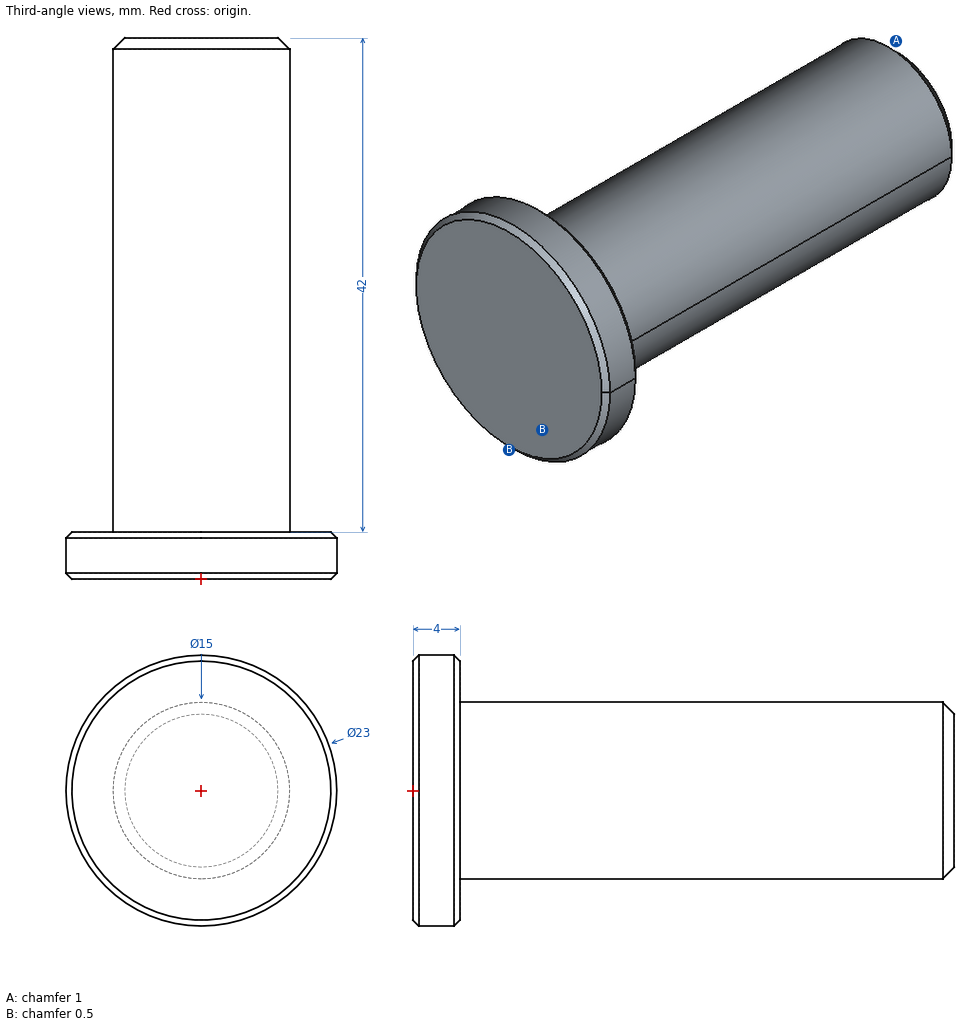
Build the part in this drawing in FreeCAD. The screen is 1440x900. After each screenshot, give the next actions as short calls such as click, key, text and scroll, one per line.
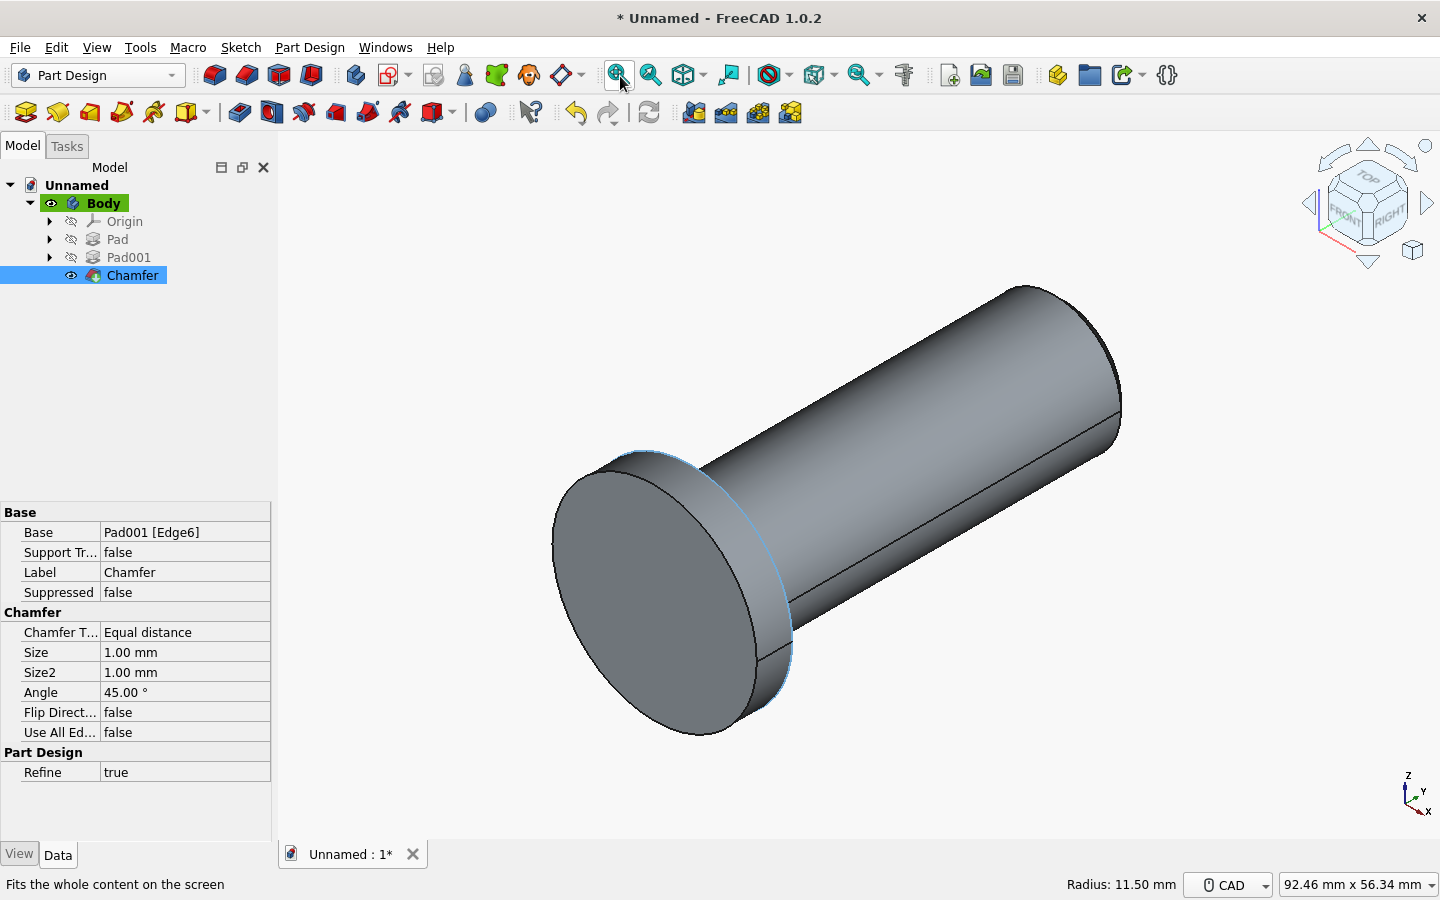
click(623, 472, ctrl)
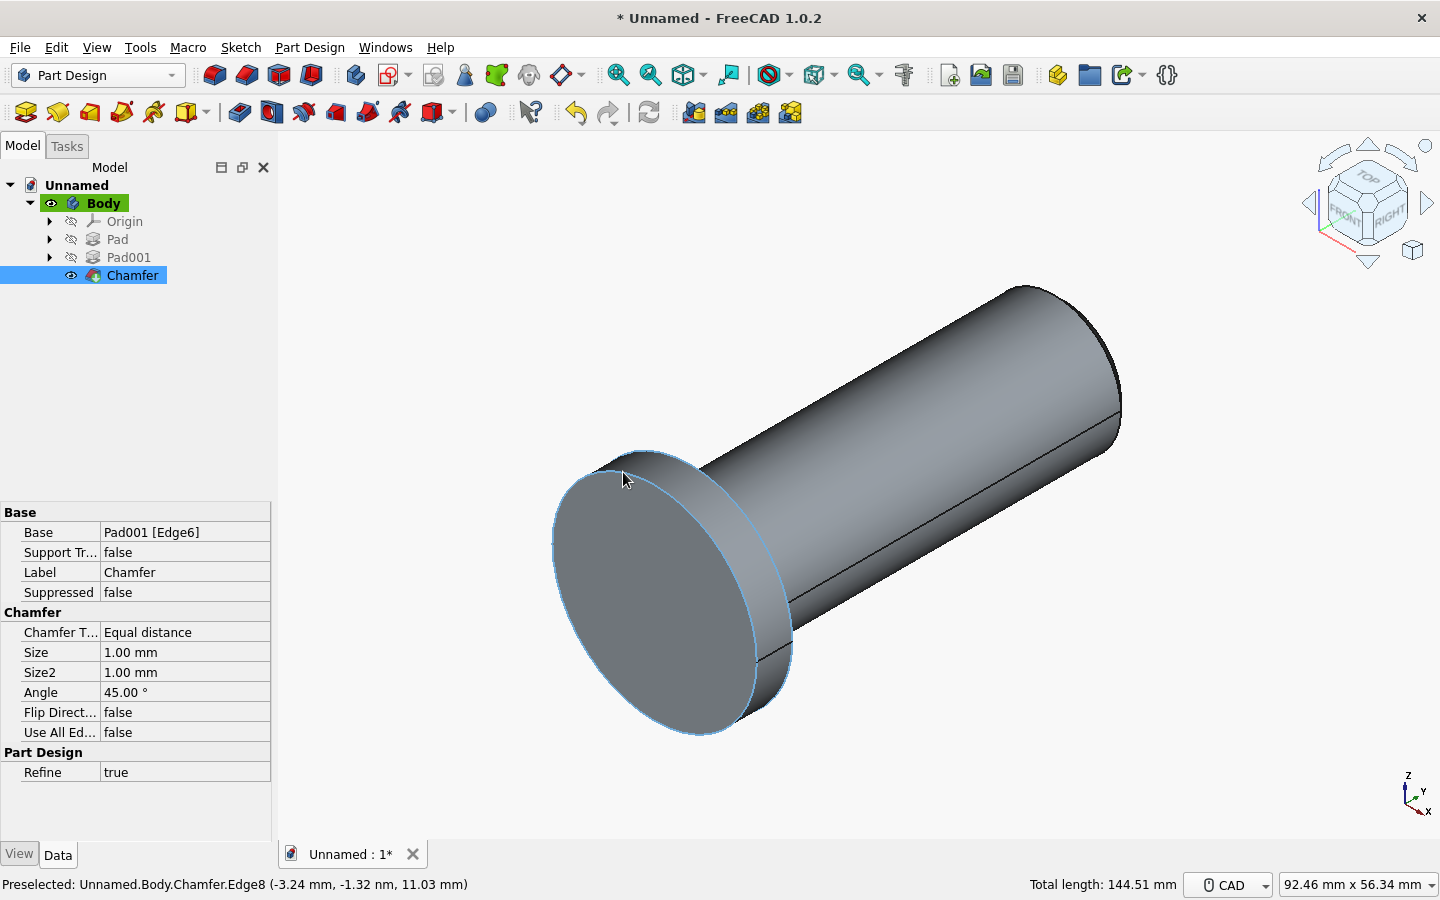
click(248, 76)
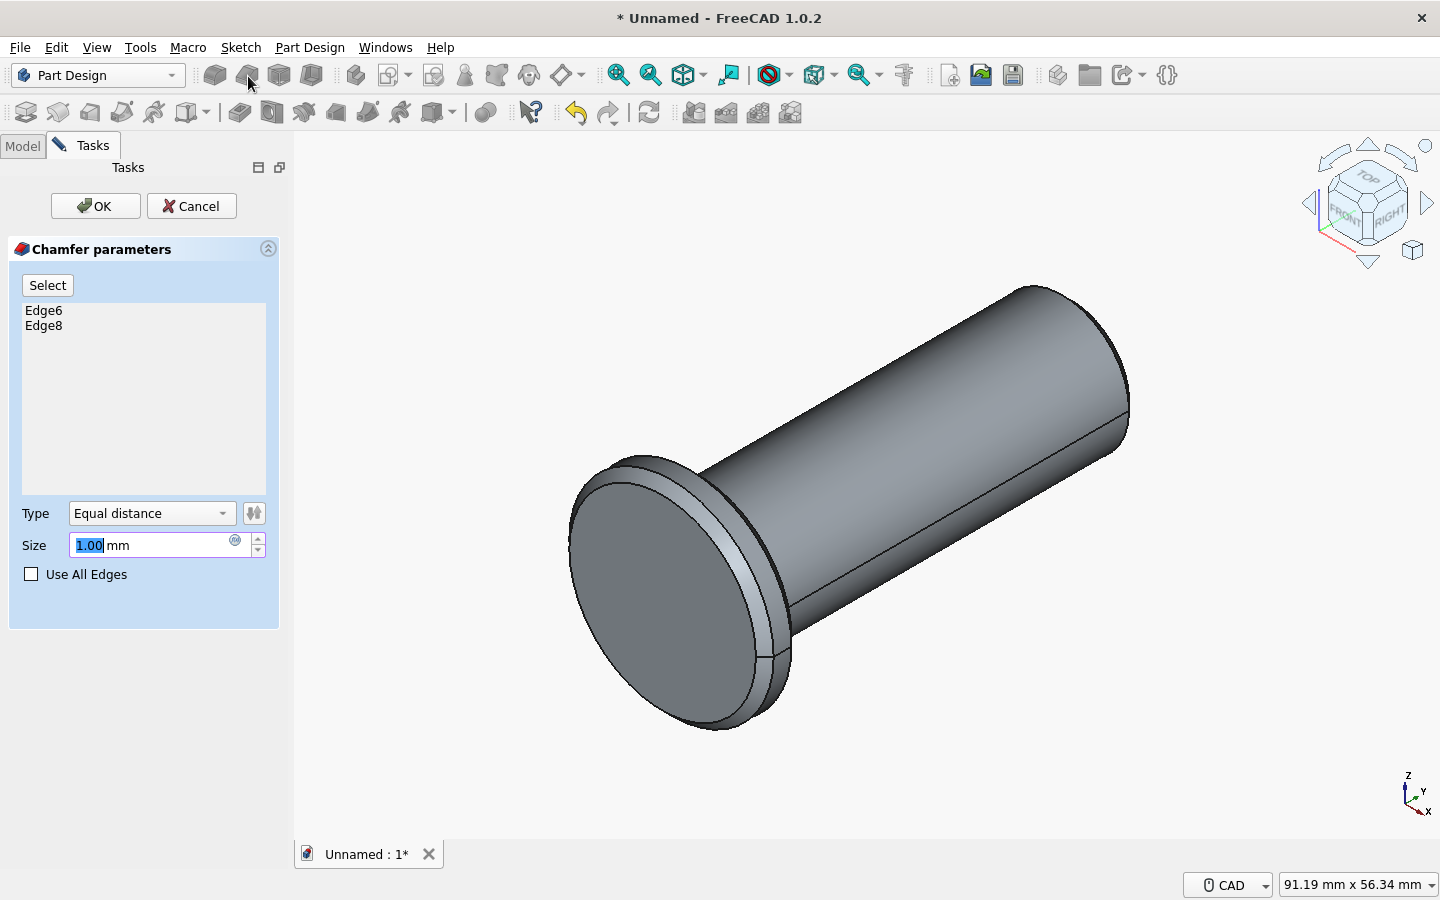
text(0.5)
key(Tab)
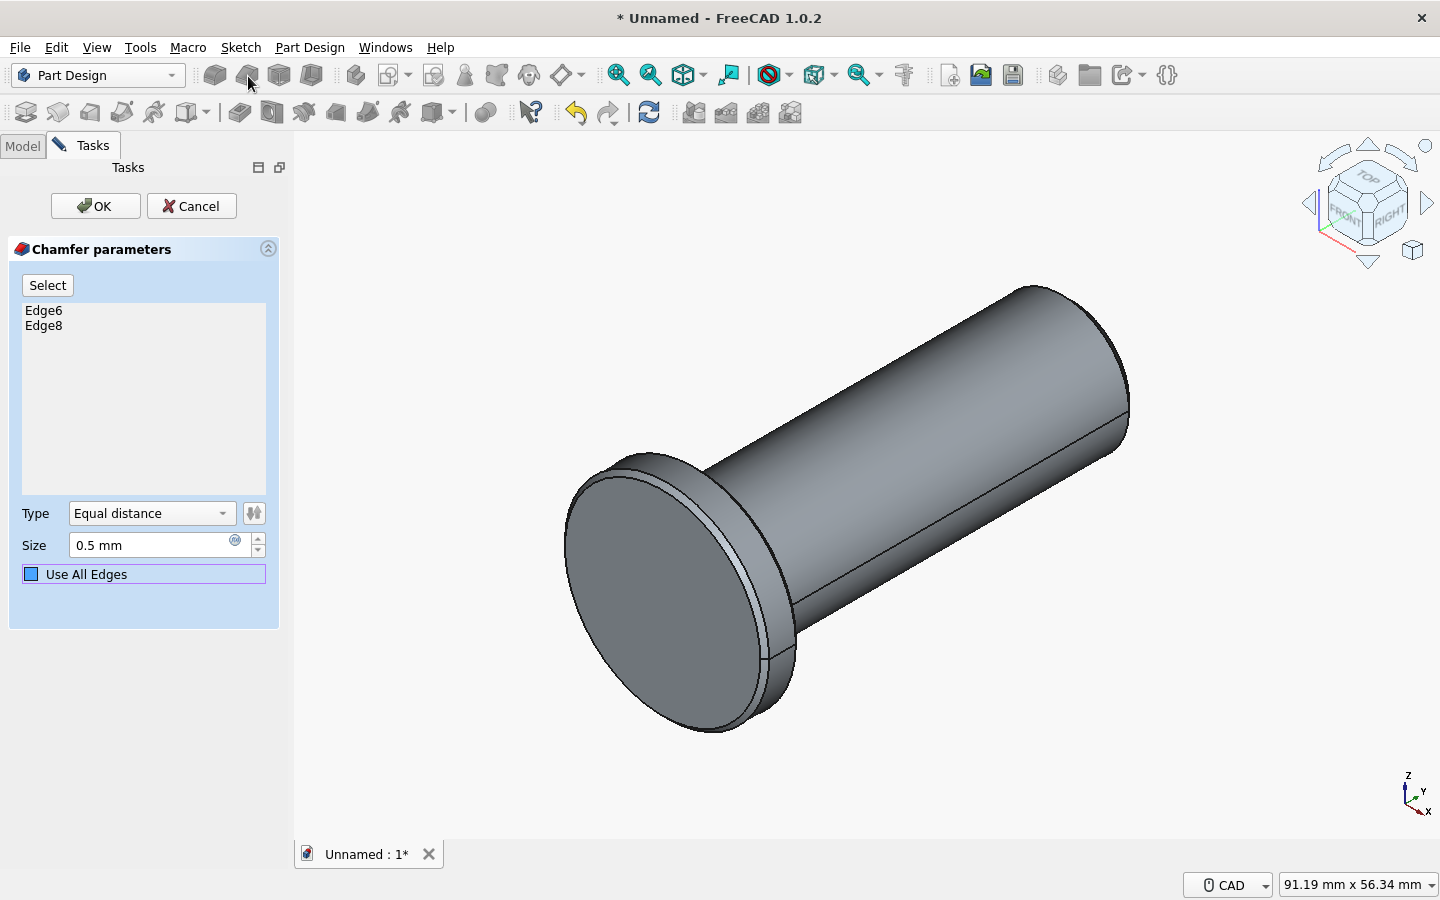
click(96, 206)